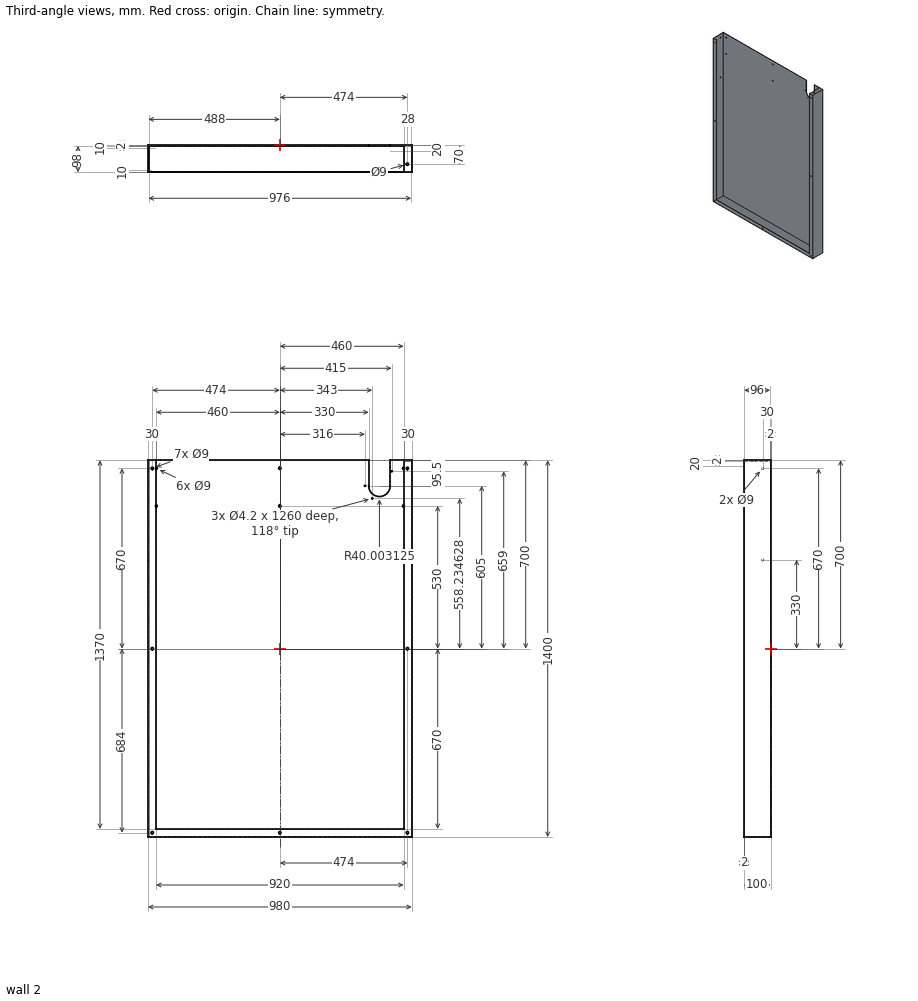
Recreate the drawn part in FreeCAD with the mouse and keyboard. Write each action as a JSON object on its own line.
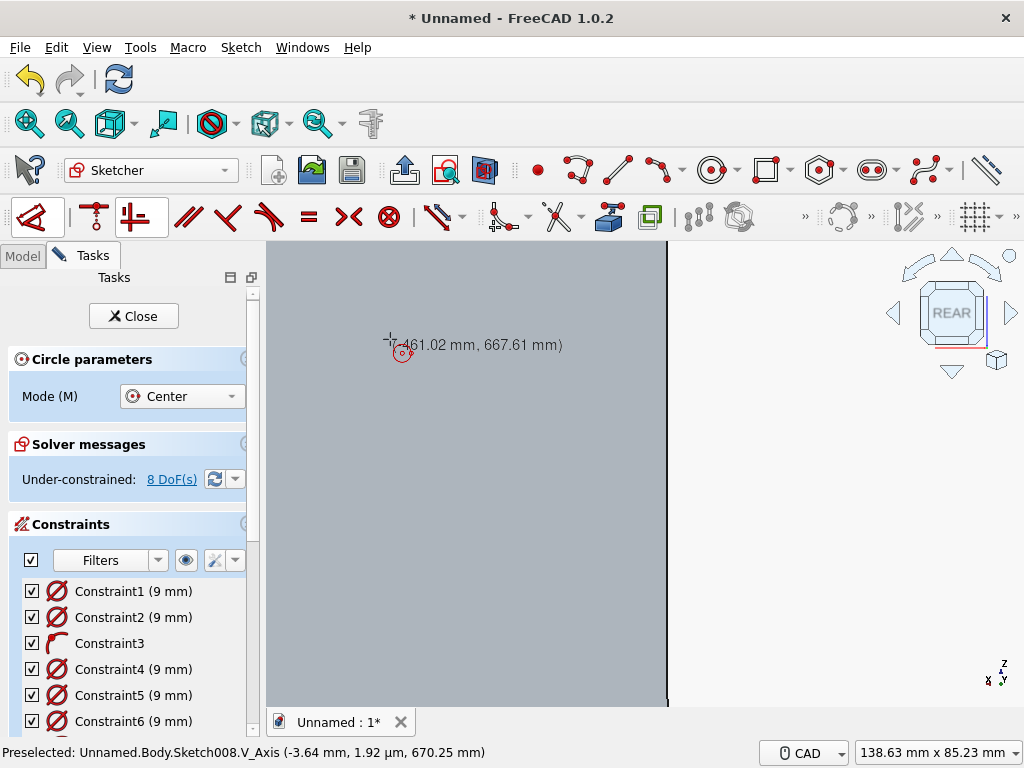
{"action": "scroll", "coordinate": [389, 339], "scroll_direction": "down", "scroll_amount": 13}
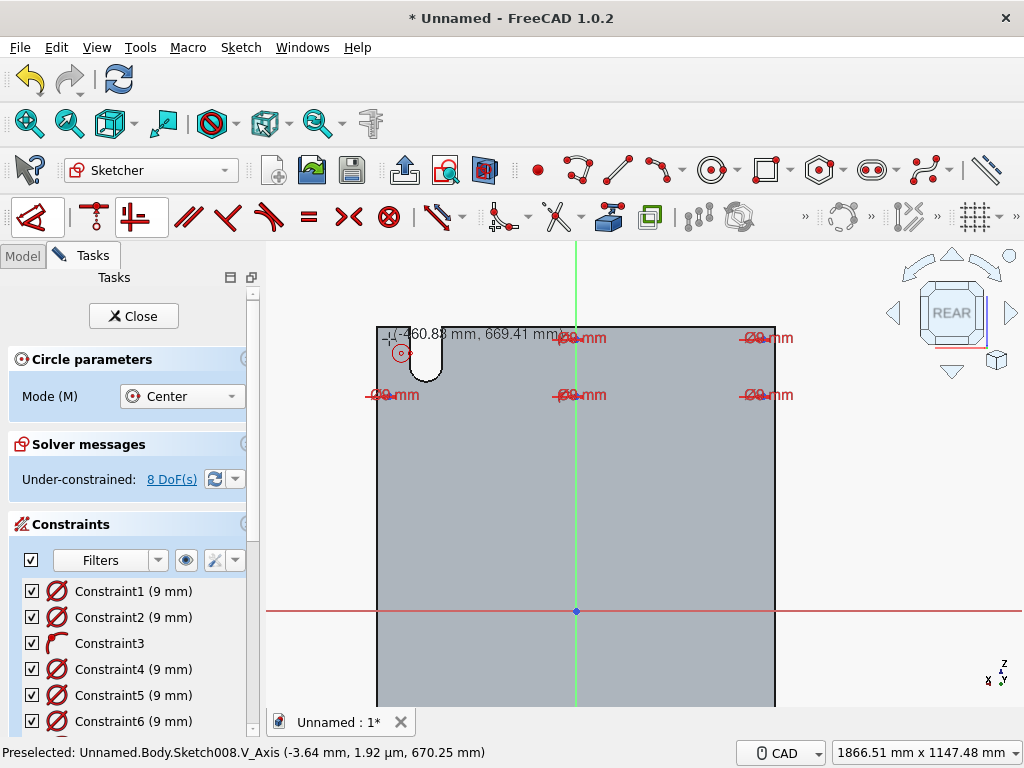
{"action": "left_click", "coordinate": [389, 339]}
{"action": "mouse_move", "coordinate": [391, 338]}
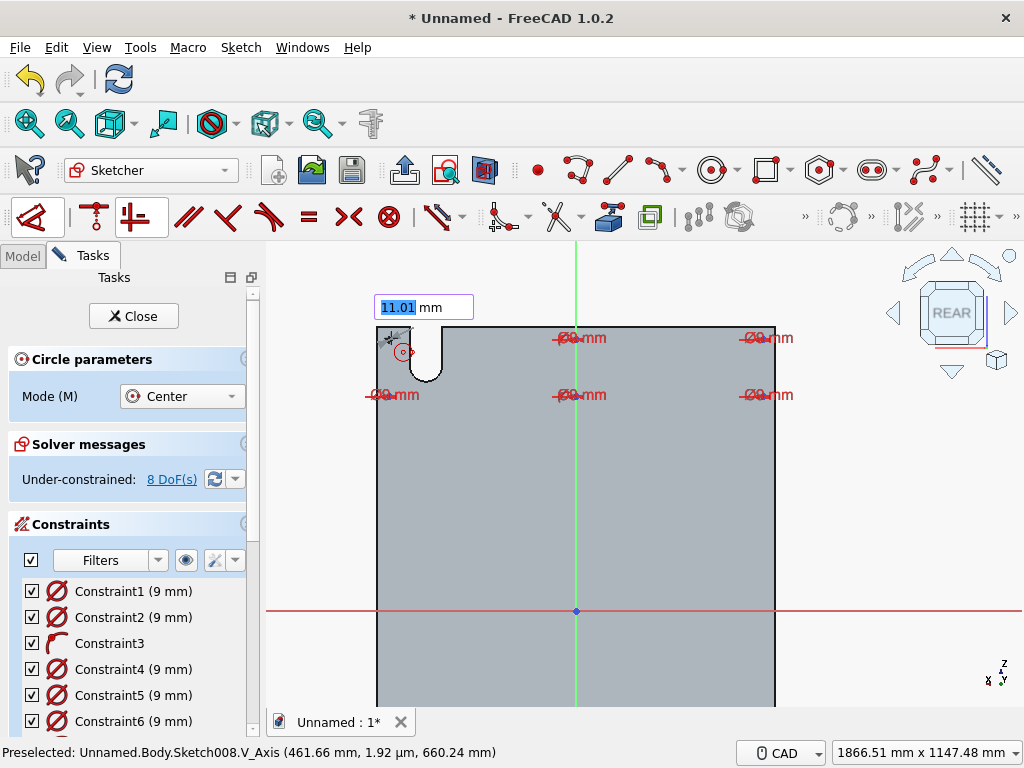
{"action": "type", "text": "9"}
{"action": "key", "text": "Return"}
{"action": "key", "text": "Escape"}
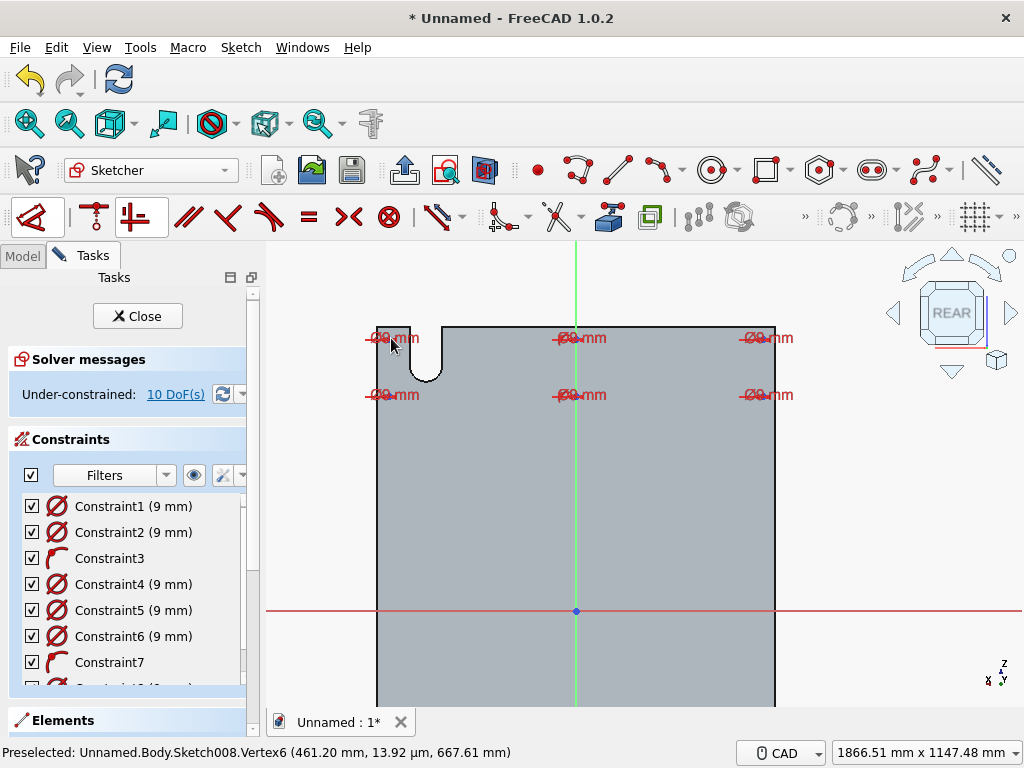
{"action": "left_click", "coordinate": [389, 397]}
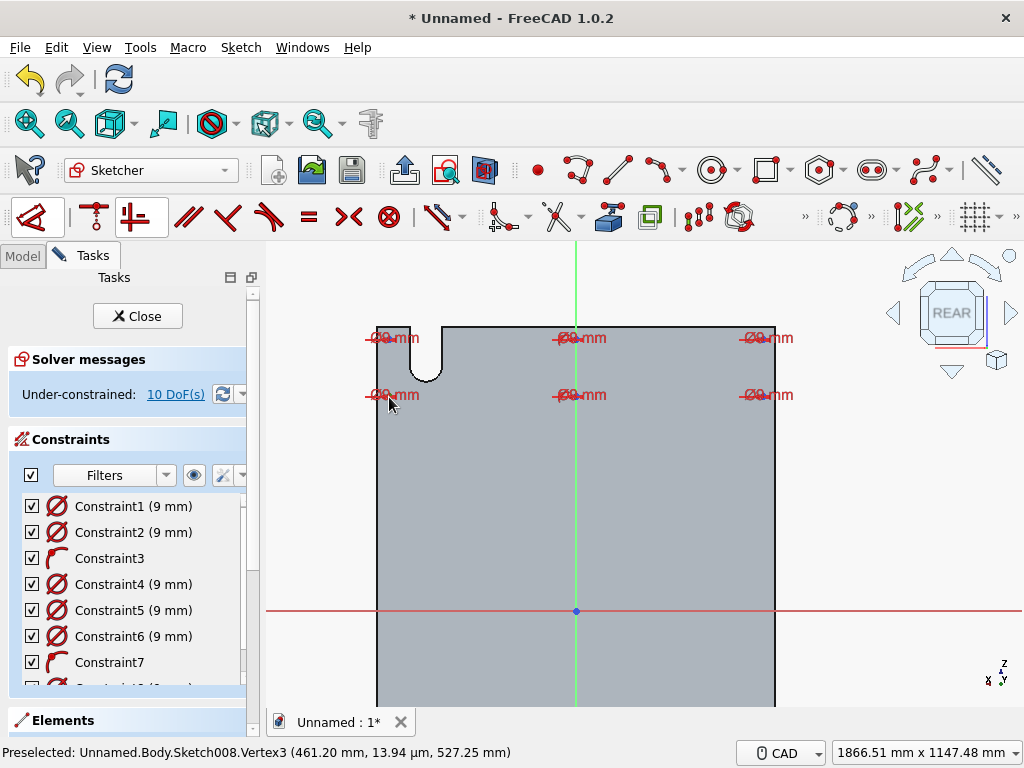
{"action": "left_click", "coordinate": [763, 397]}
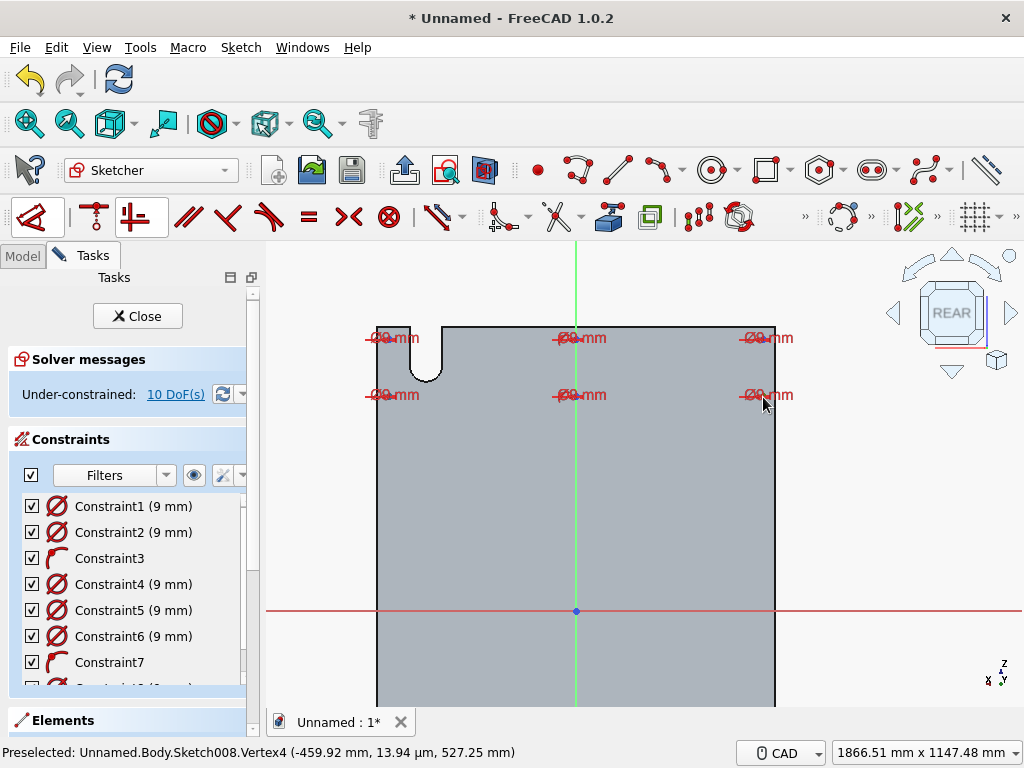
{"action": "left_click", "coordinate": [576, 650]}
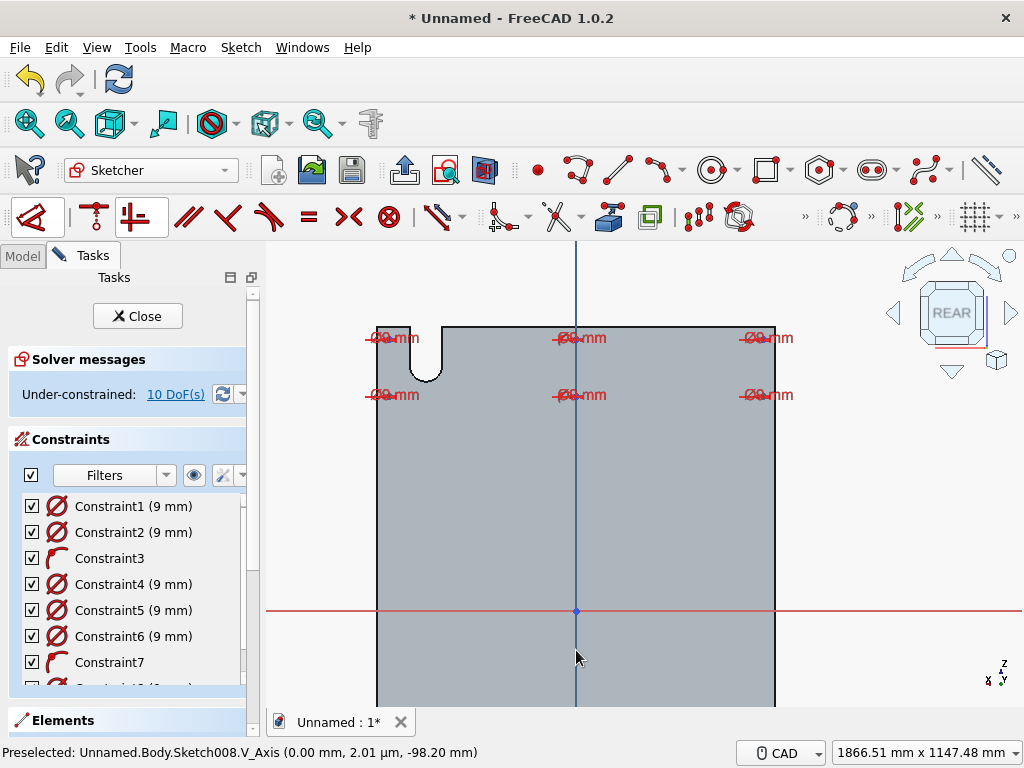
{"action": "left_click", "coordinate": [350, 218]}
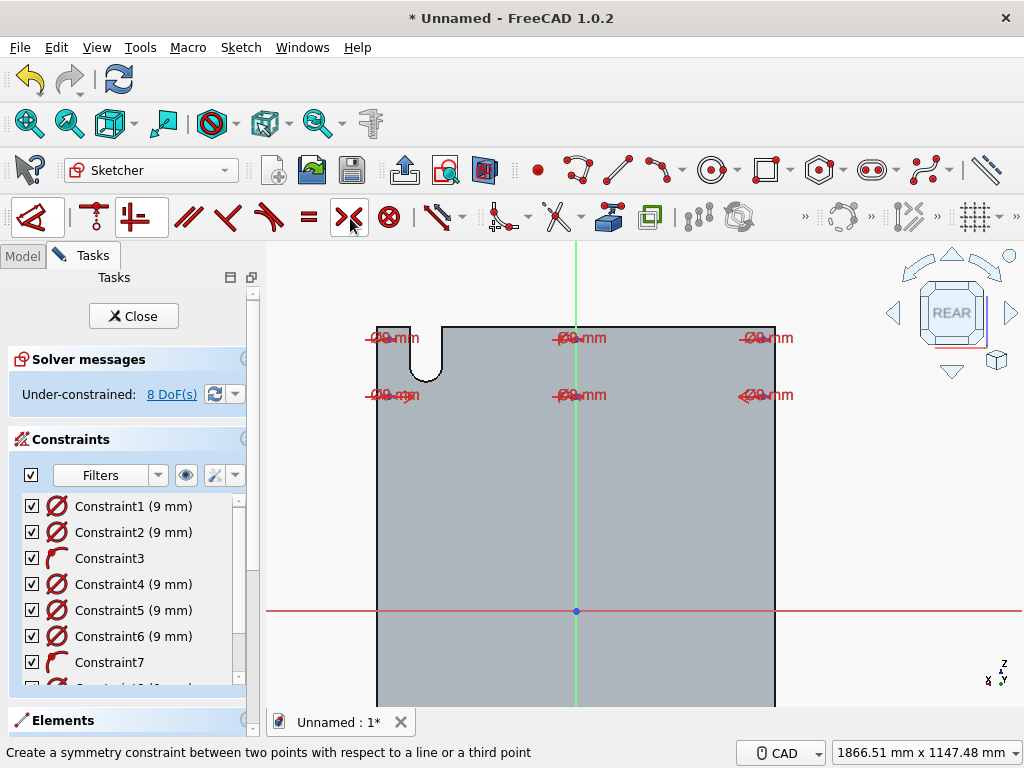
{"action": "left_click", "coordinate": [763, 340]}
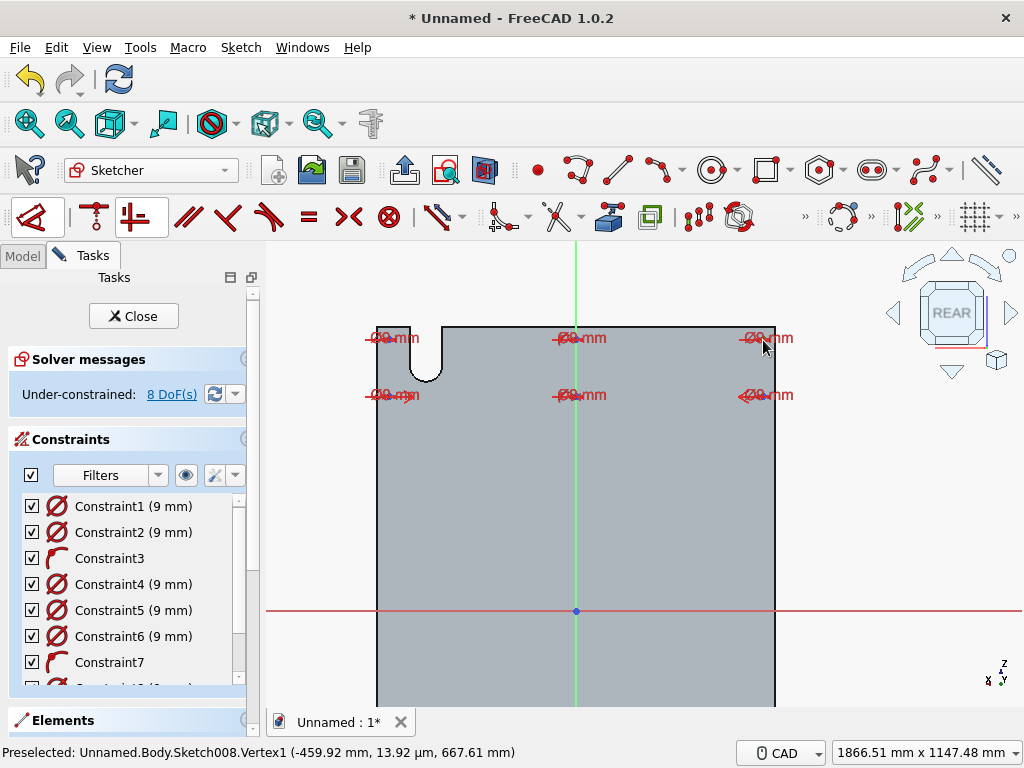
{"action": "left_click", "coordinate": [389, 340]}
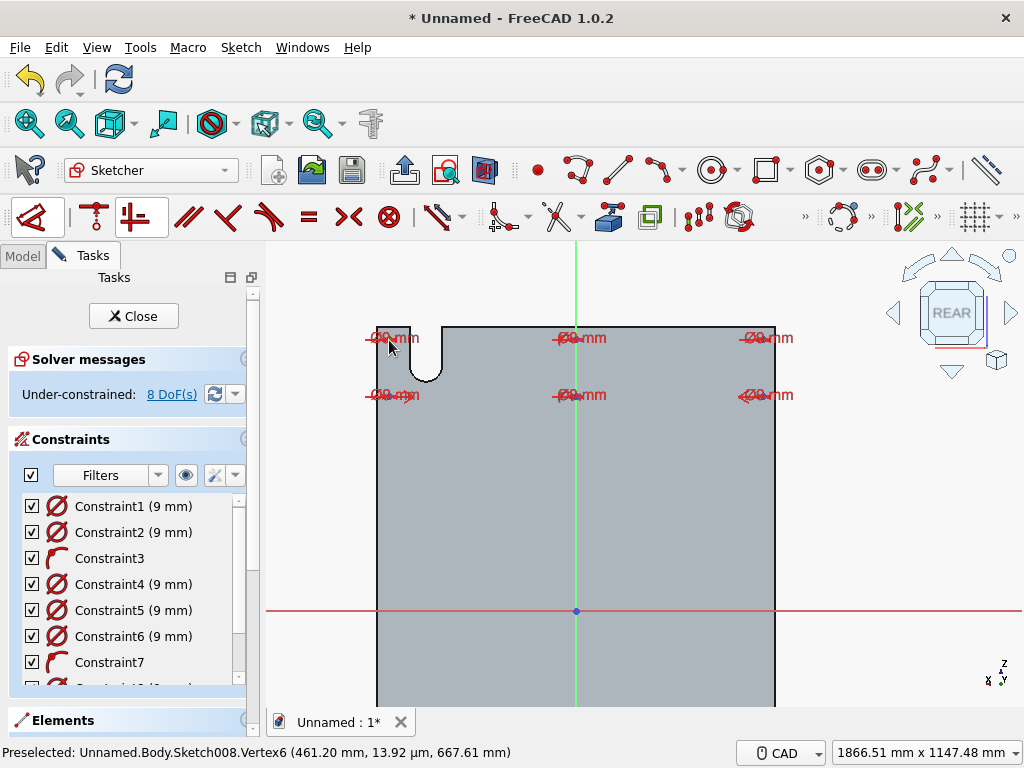
{"action": "left_click", "coordinate": [576, 650]}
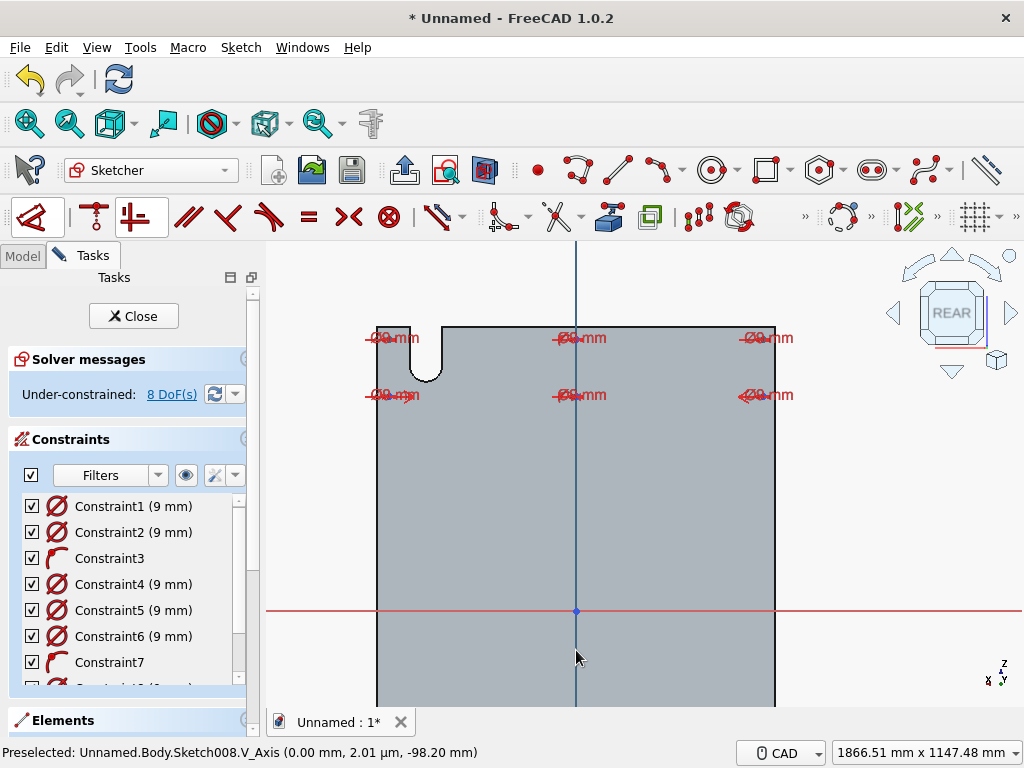
{"action": "left_click", "coordinate": [350, 218]}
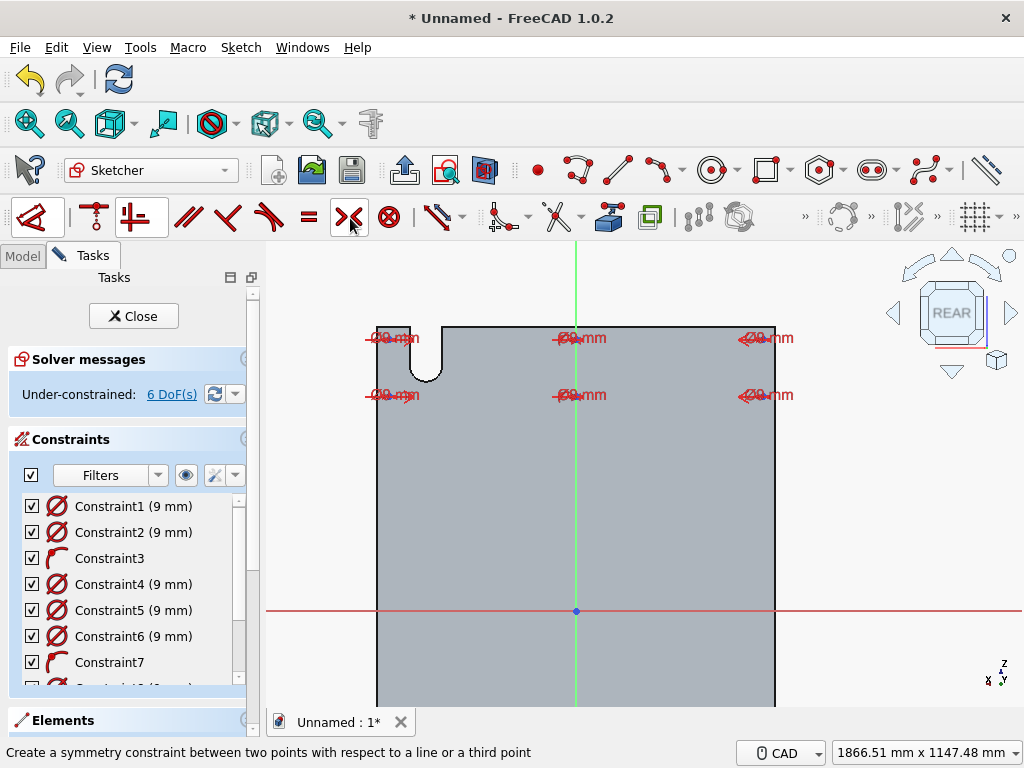
{"action": "left_click", "coordinate": [763, 340]}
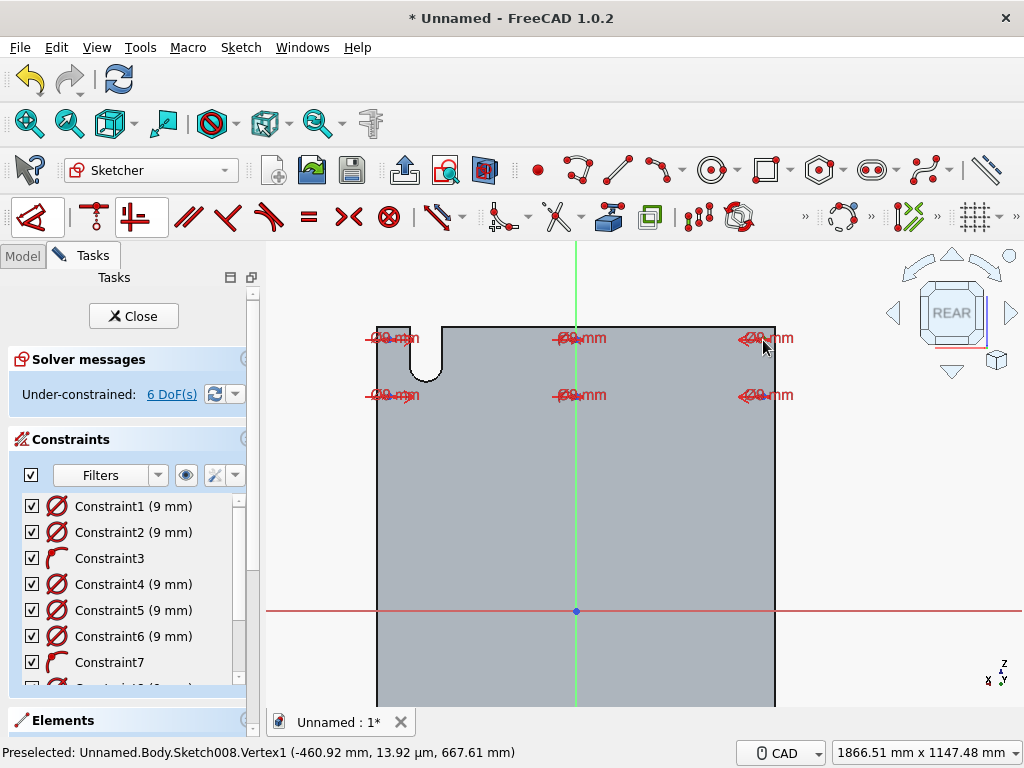
{"action": "key", "text": "l"}